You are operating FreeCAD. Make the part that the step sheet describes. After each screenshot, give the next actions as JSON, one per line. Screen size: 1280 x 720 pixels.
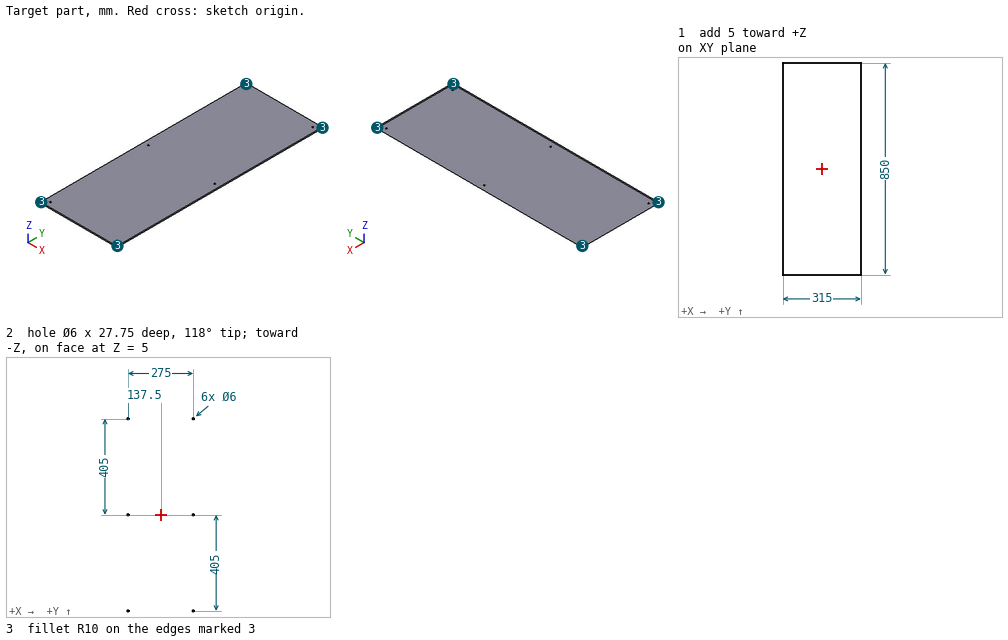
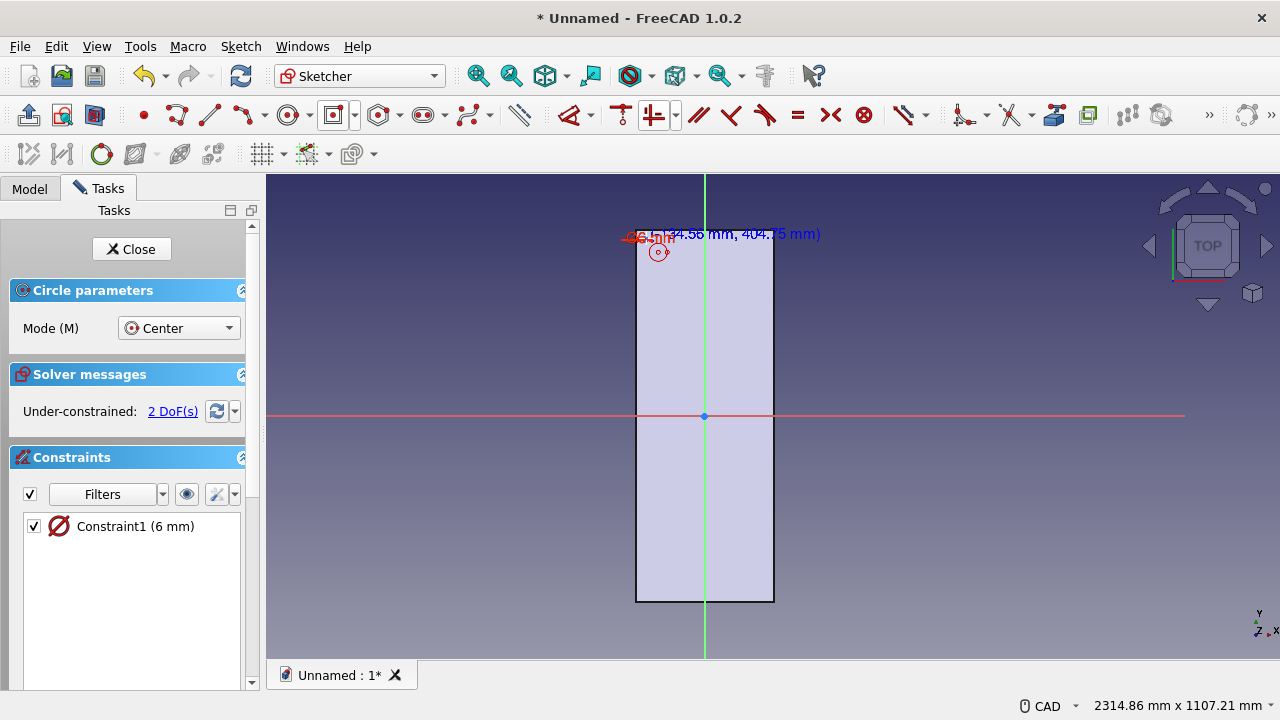
{"action": "scroll", "coordinate": [765, 239], "scroll_direction": "up", "scroll_amount": 15}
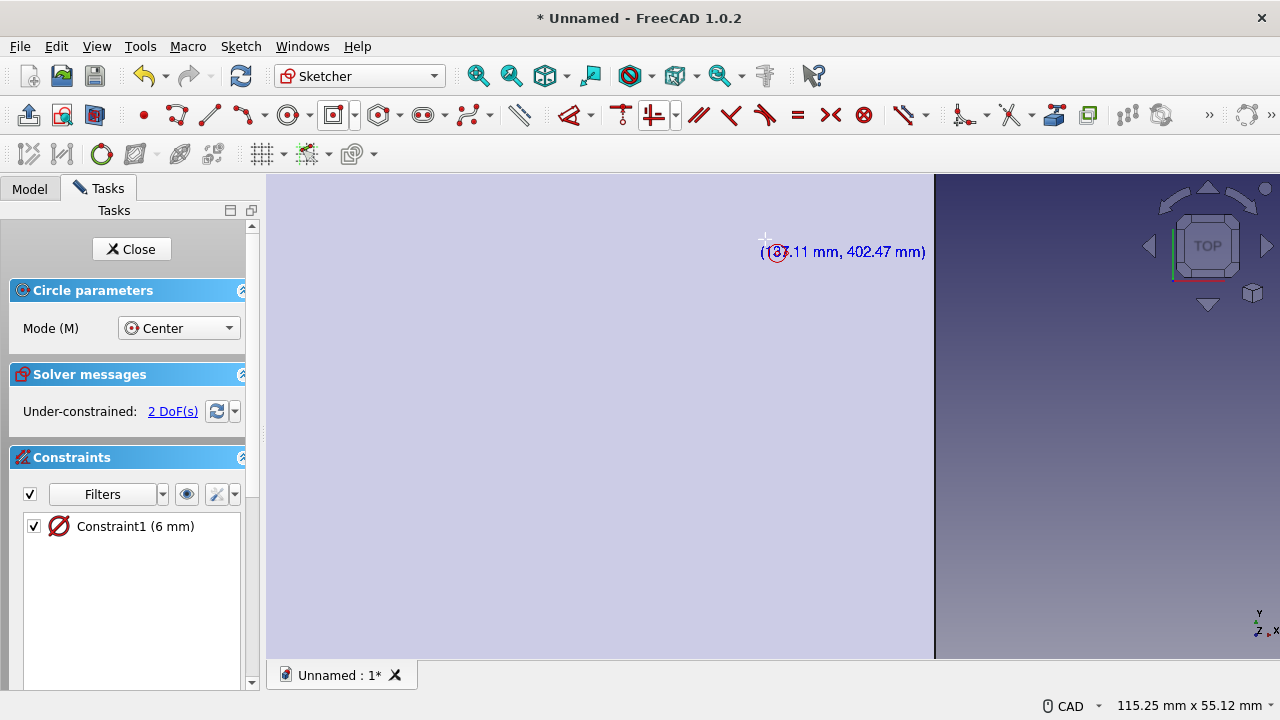
{"action": "scroll", "coordinate": [765, 239], "scroll_direction": "down", "scroll_amount": 15}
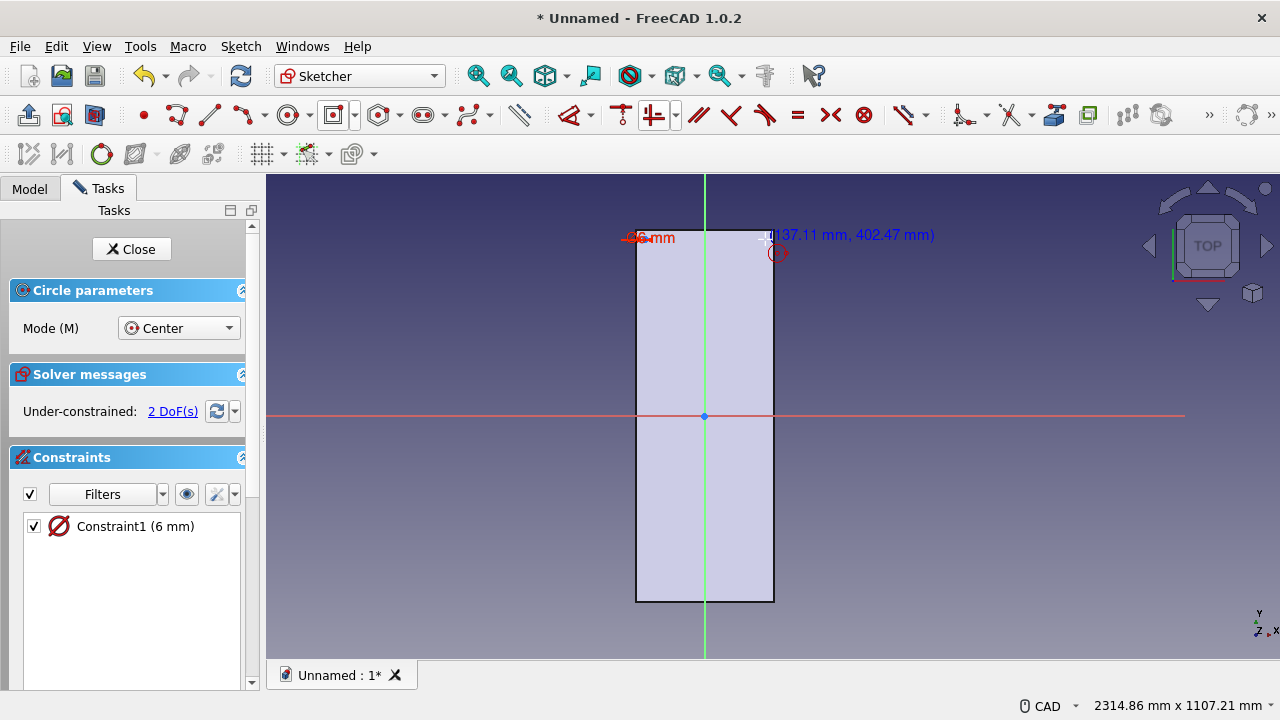
{"action": "left_click", "coordinate": [765, 239]}
{"action": "mouse_move", "coordinate": [766, 238]}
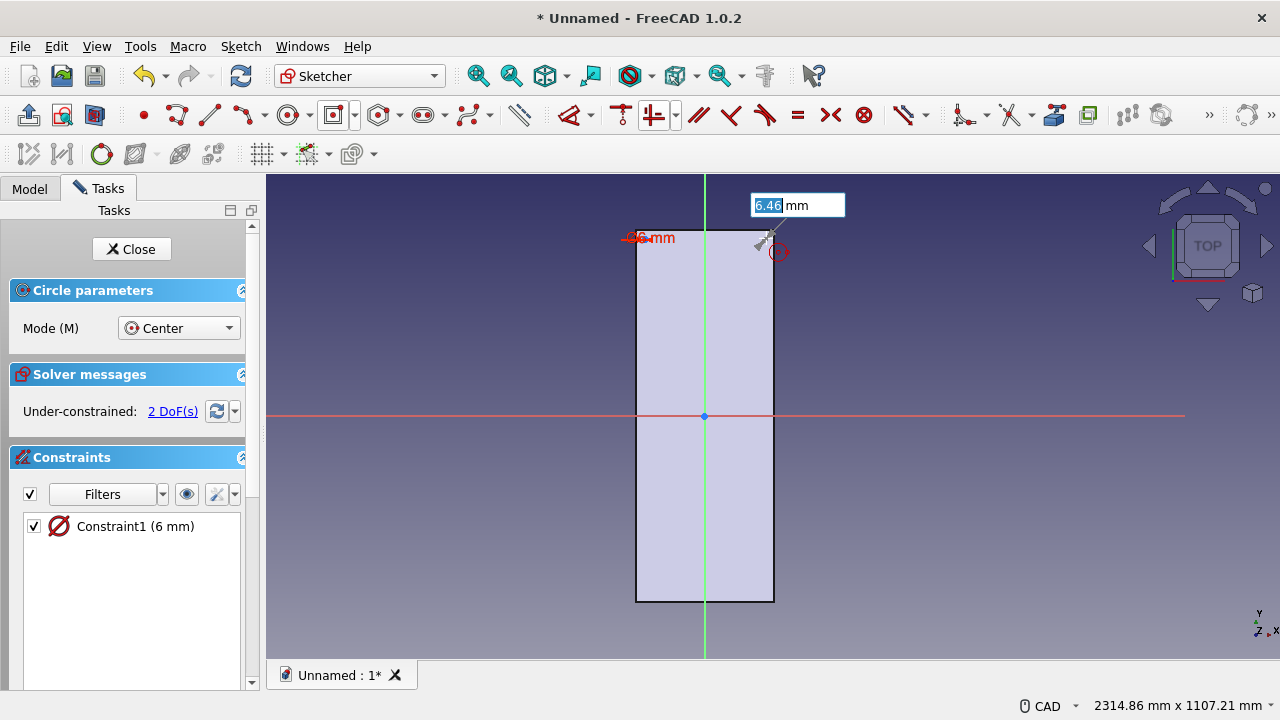
{"action": "type", "text": "6"}
{"action": "key", "text": "Return"}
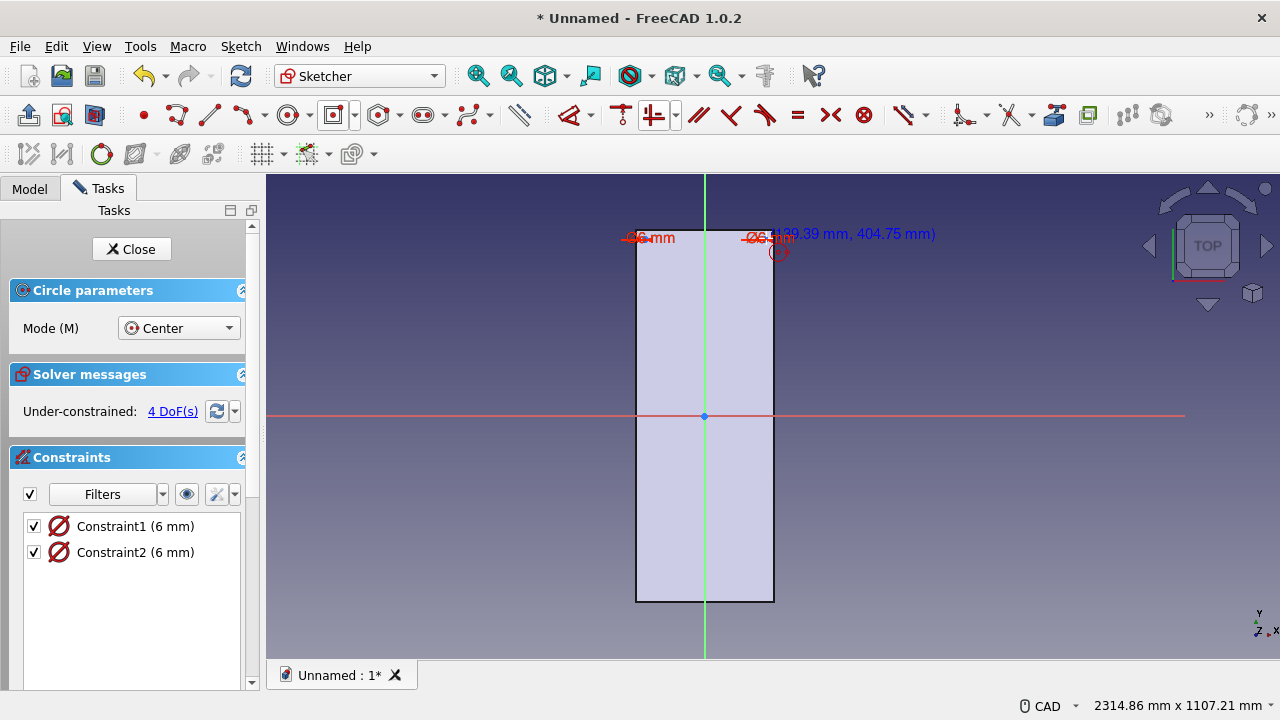
{"action": "scroll", "coordinate": [765, 594], "scroll_direction": "up", "scroll_amount": 15}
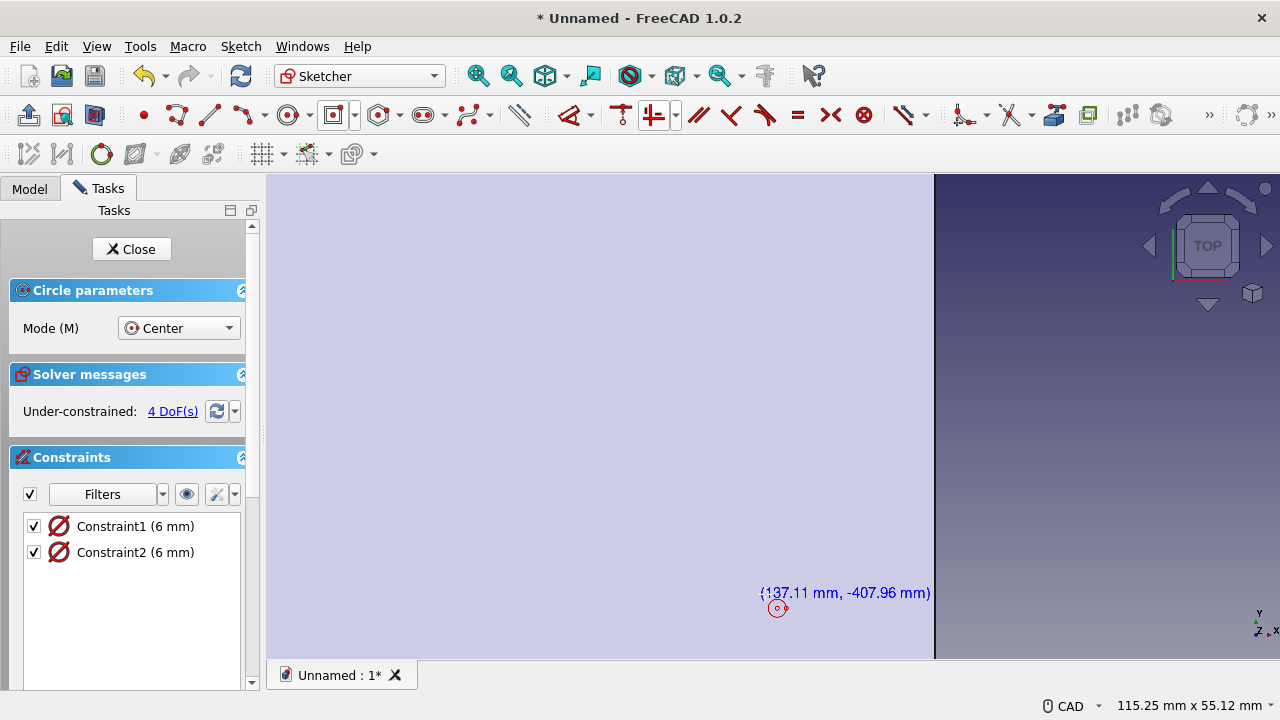
{"action": "scroll", "coordinate": [765, 595], "scroll_direction": "down", "scroll_amount": 15}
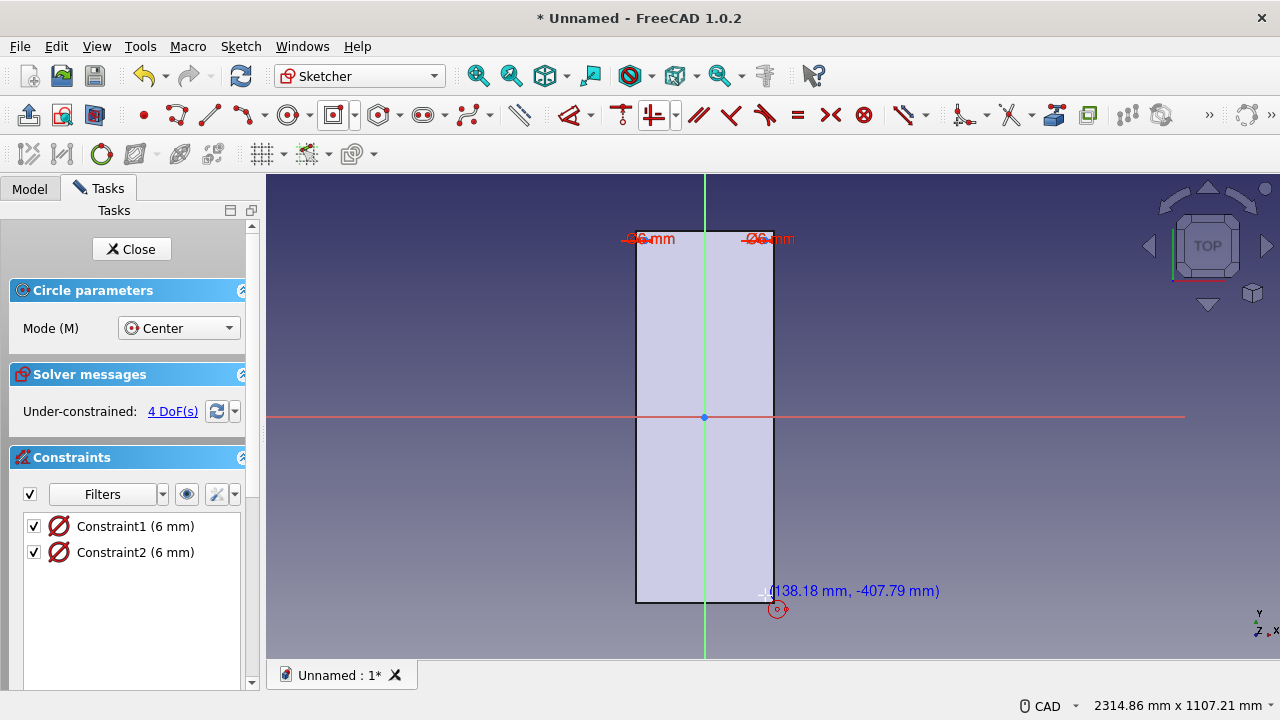
{"action": "left_click", "coordinate": [765, 595]}
{"action": "mouse_move", "coordinate": [766, 594]}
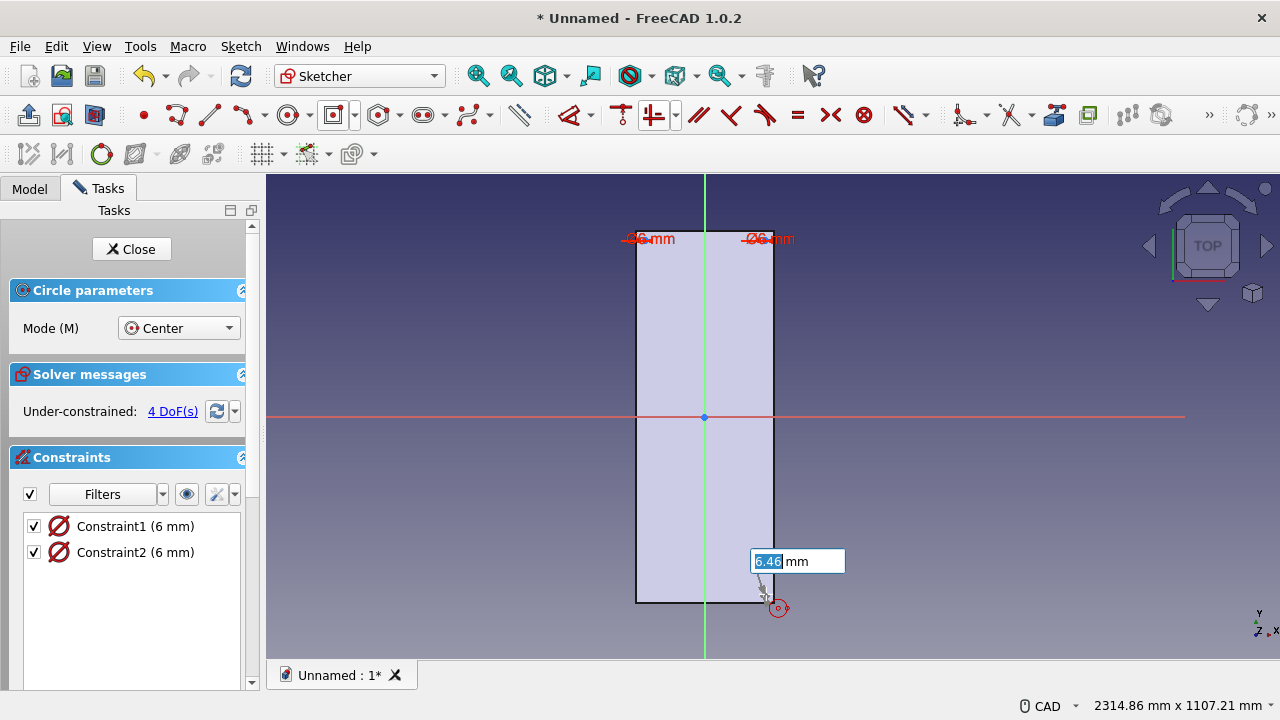
{"action": "type", "text": "6"}
{"action": "key", "text": "Return"}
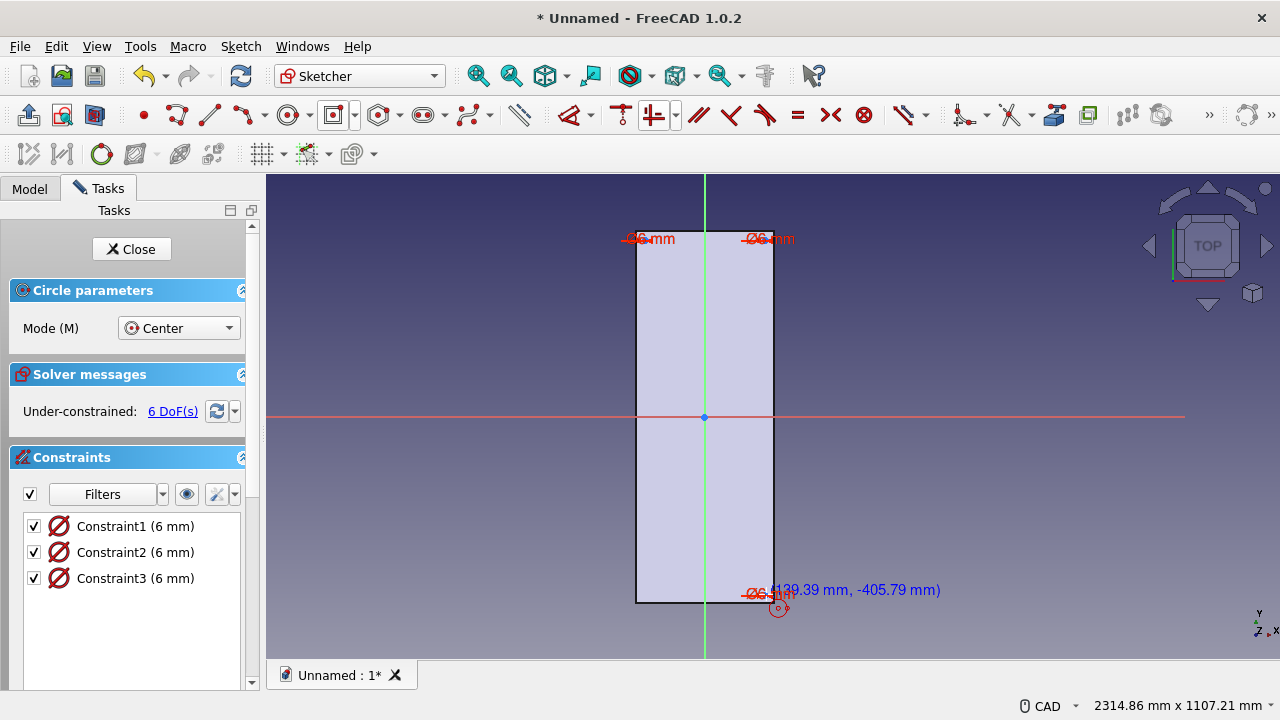
{"action": "scroll", "coordinate": [645, 595], "scroll_direction": "up", "scroll_amount": 15}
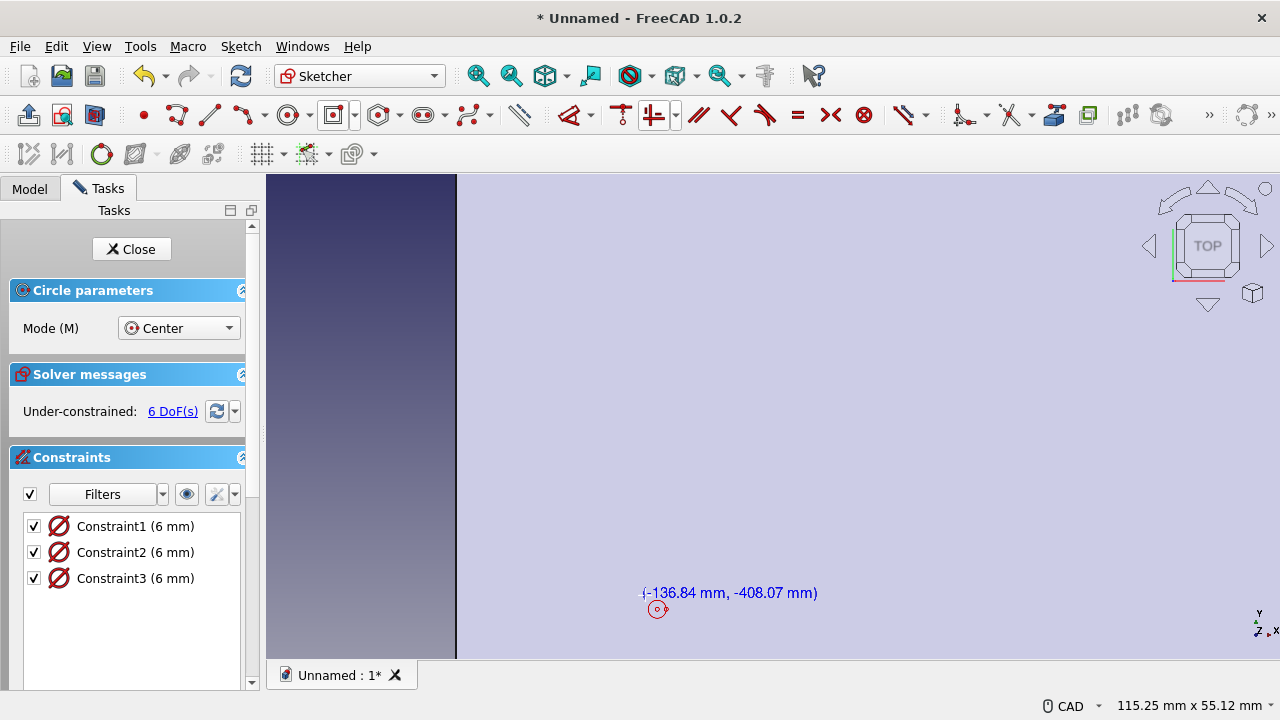
{"action": "scroll", "coordinate": [645, 595], "scroll_direction": "down", "scroll_amount": 15}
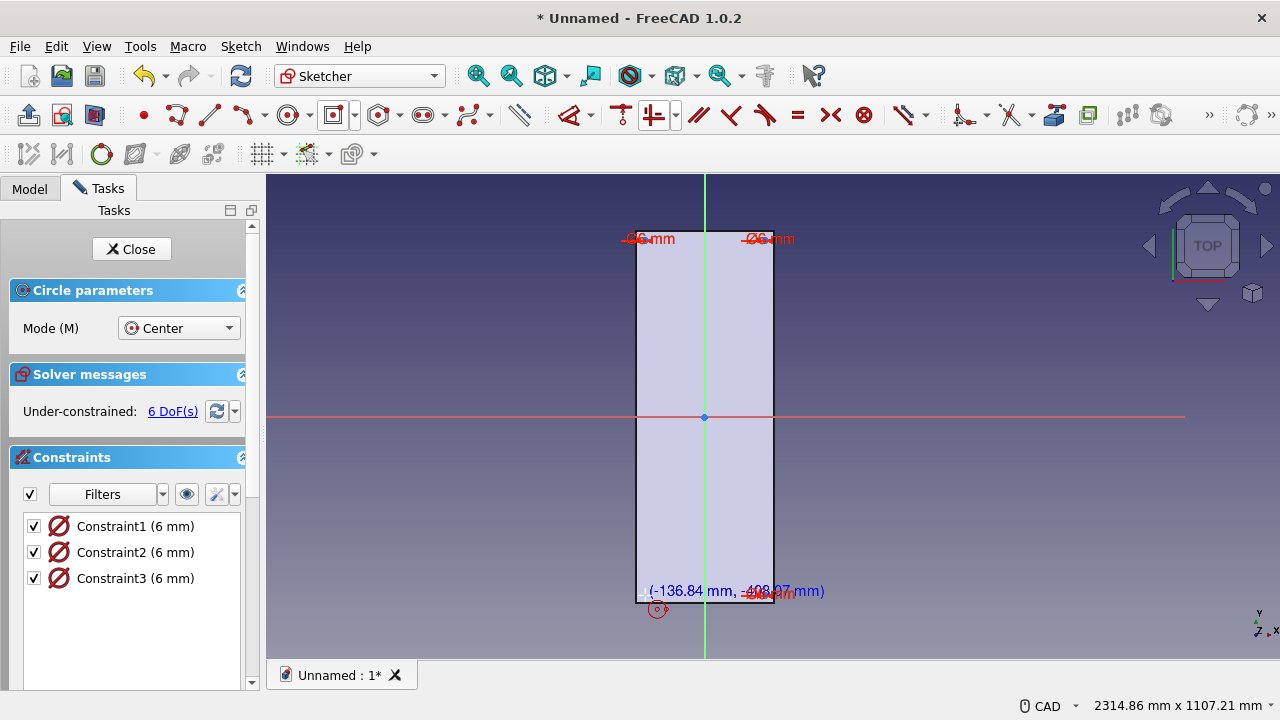
{"action": "left_click", "coordinate": [645, 595]}
{"action": "mouse_move", "coordinate": [646, 594]}